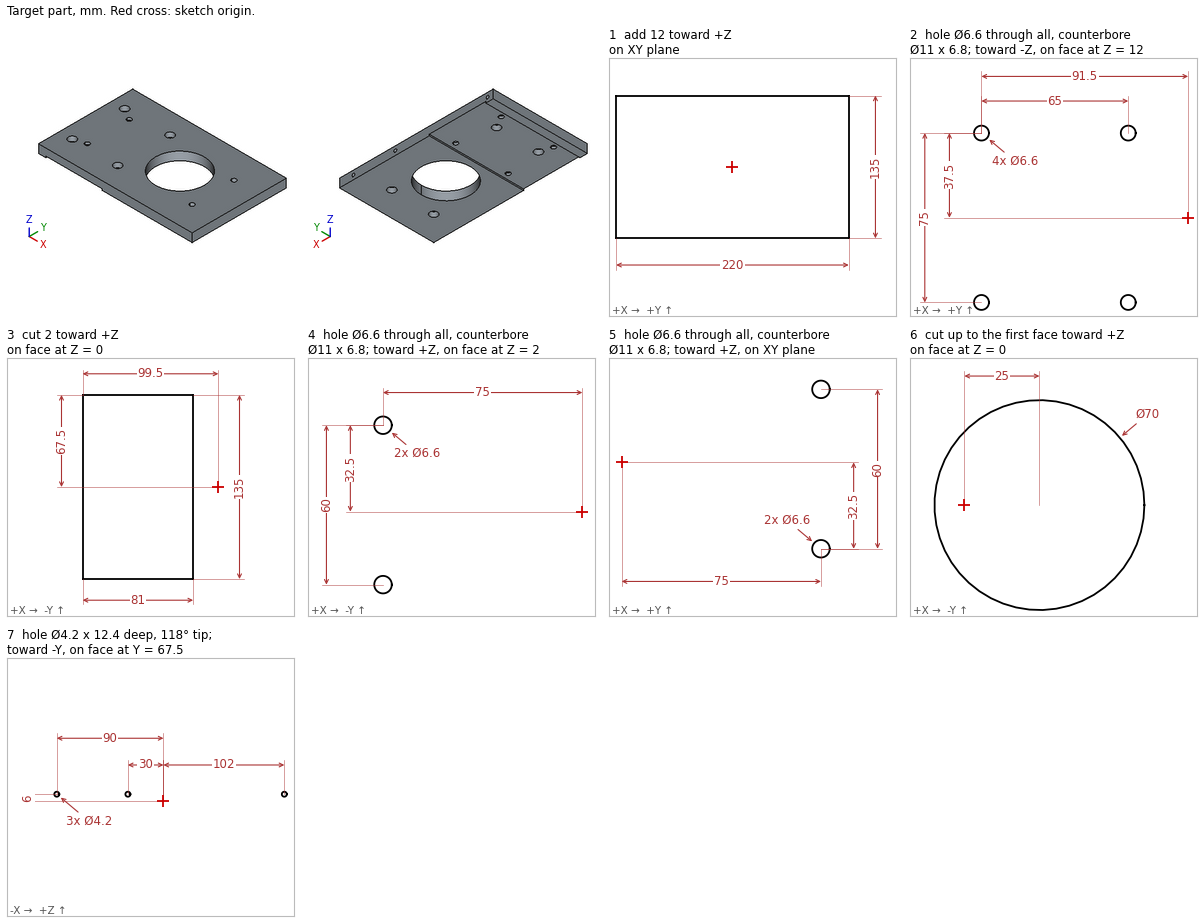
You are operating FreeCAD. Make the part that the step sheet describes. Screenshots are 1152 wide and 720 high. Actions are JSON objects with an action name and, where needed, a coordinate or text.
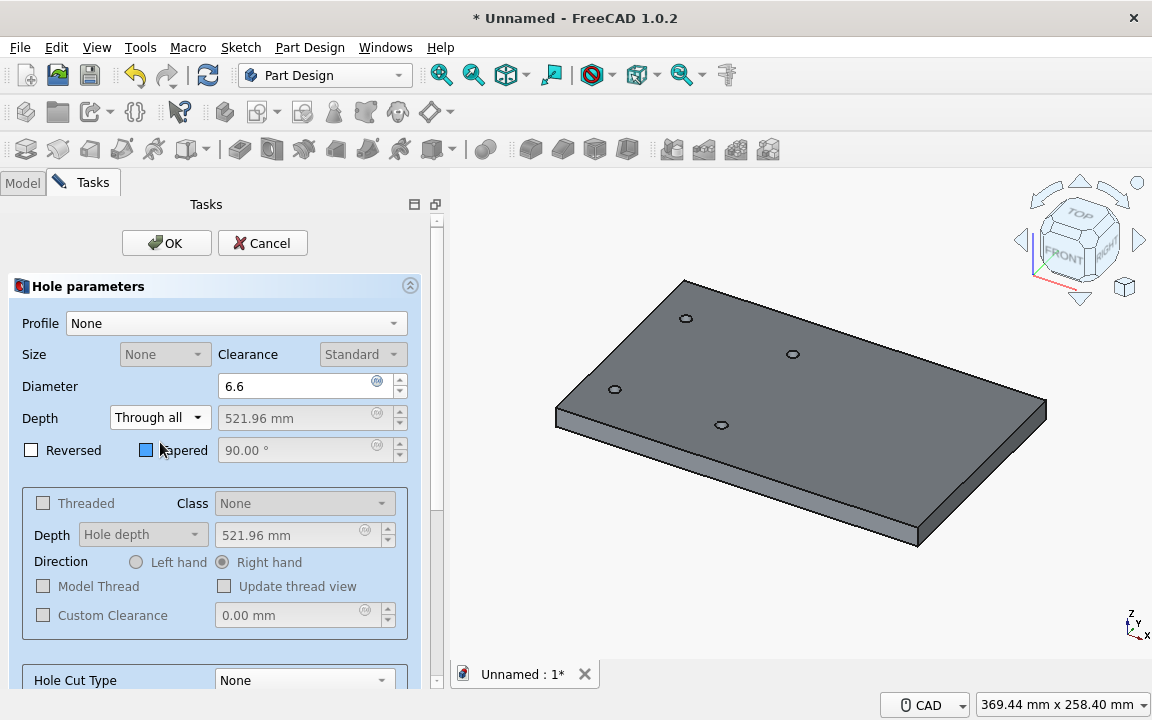
{"action": "scroll", "coordinate": [437, 451], "scroll_direction": "down", "scroll_amount": 2}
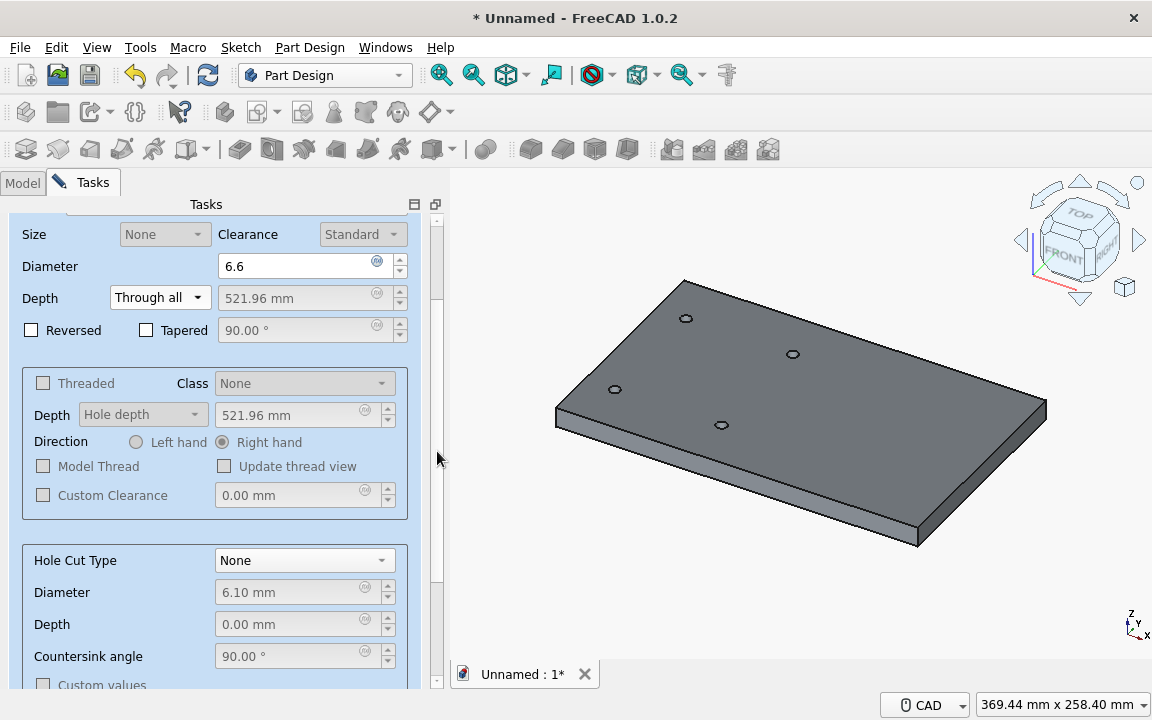
{"action": "left_click", "coordinate": [306, 560]}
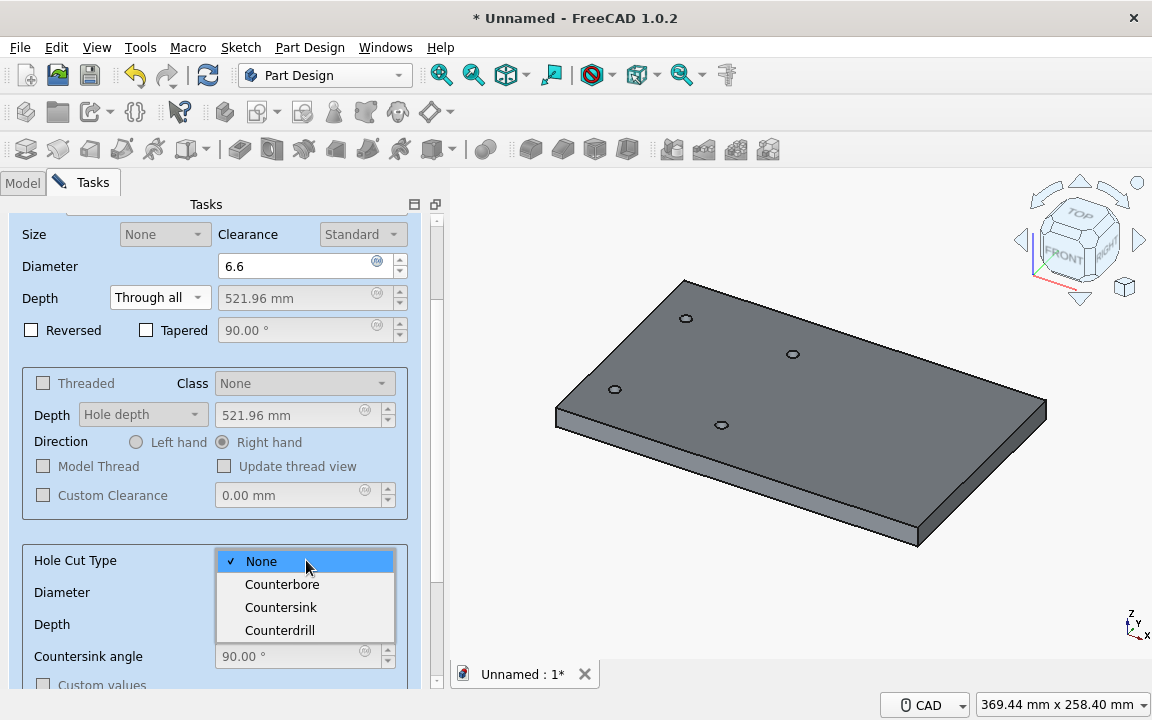
{"action": "left_click", "coordinate": [304, 584]}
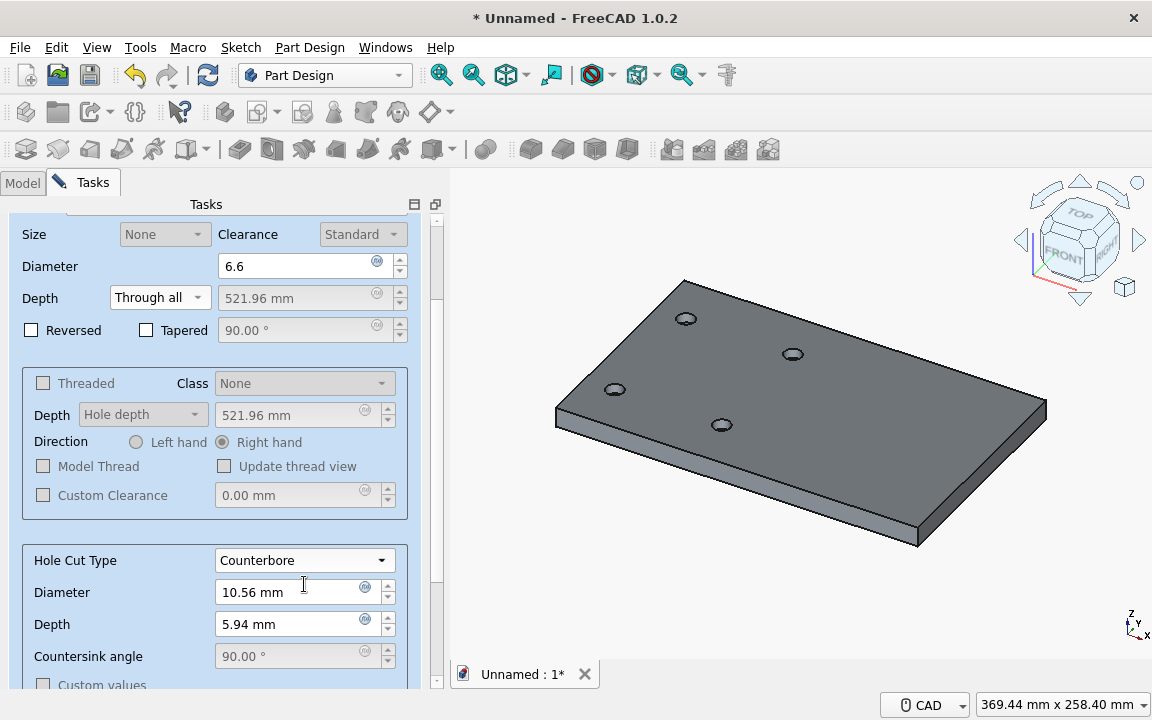
{"action": "triple_click", "coordinate": [298, 592]}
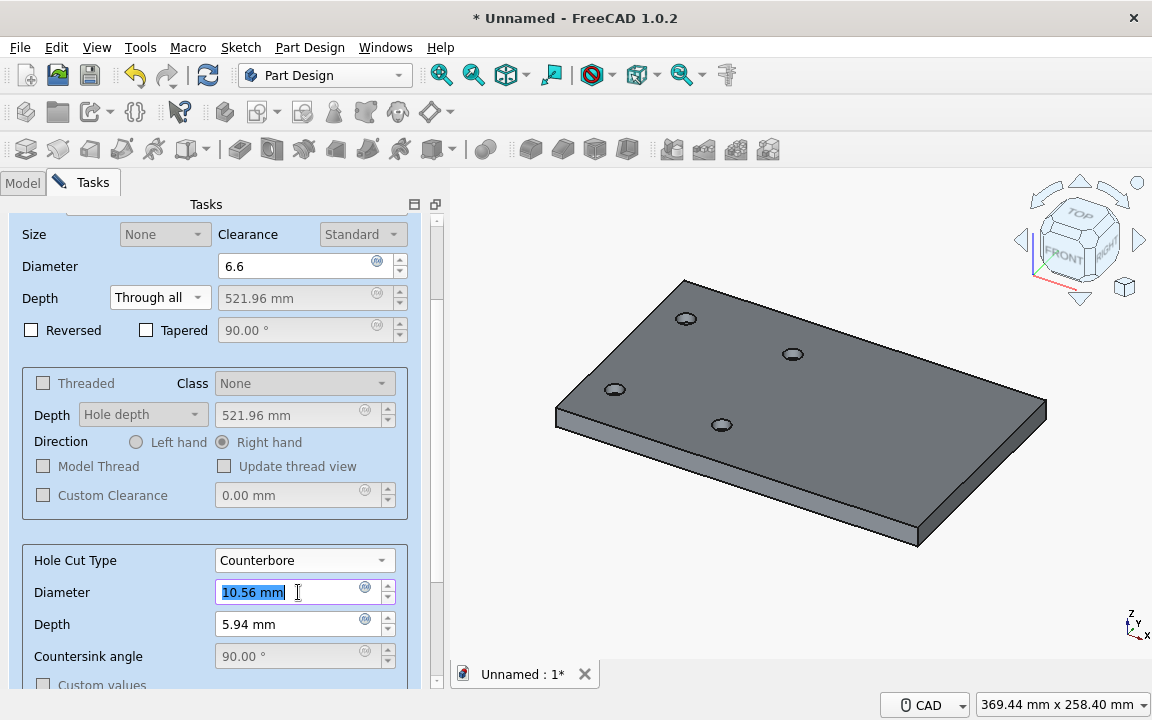
{"action": "type", "text": "11"}
{"action": "key", "text": "Tab"}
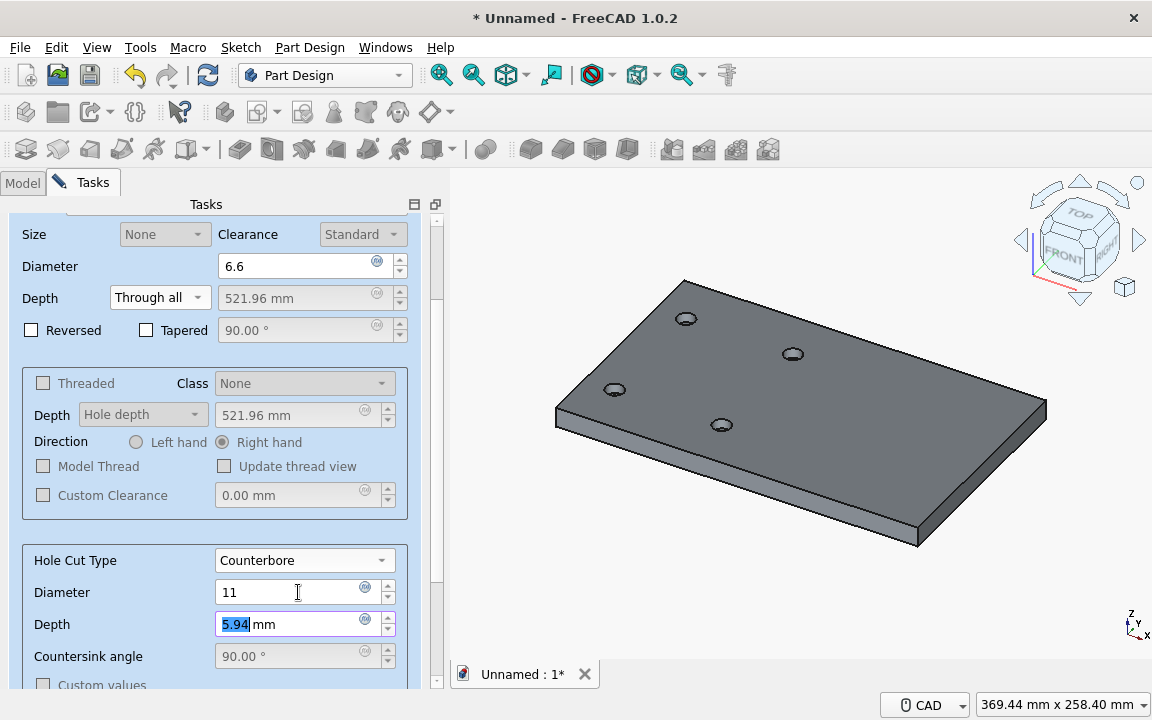
{"action": "type", "text": "6.8"}
{"action": "key", "text": "Tab"}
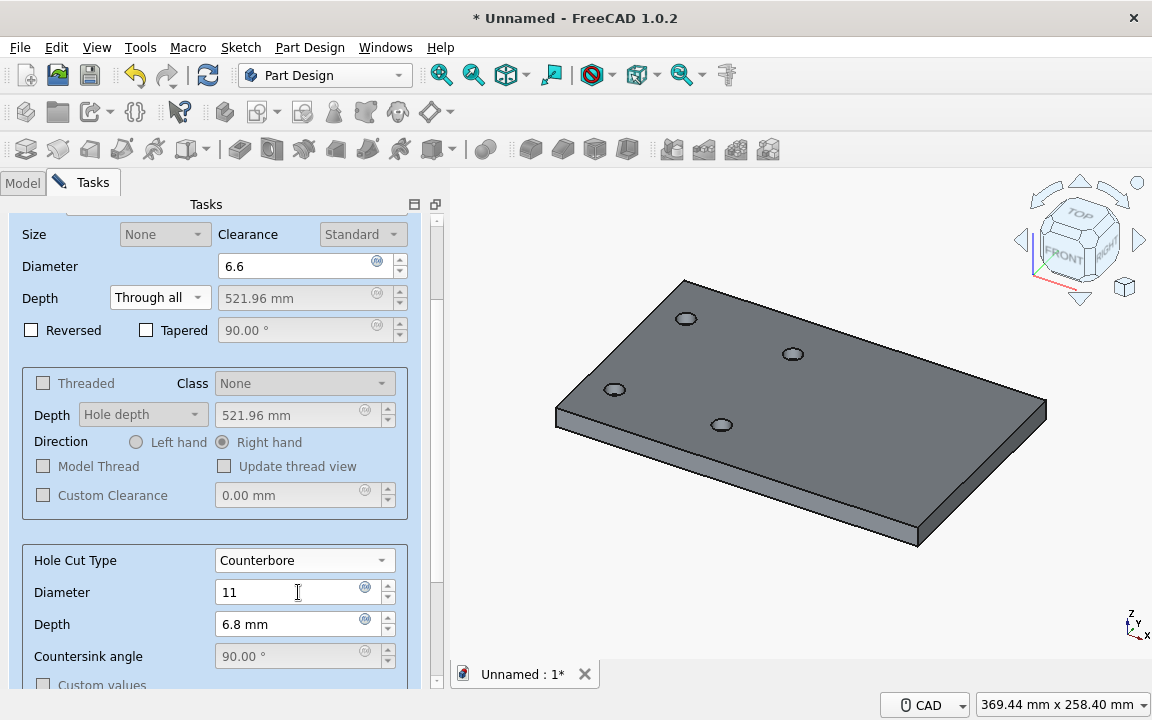
{"action": "scroll", "coordinate": [437, 451], "scroll_direction": "up", "scroll_amount": 3}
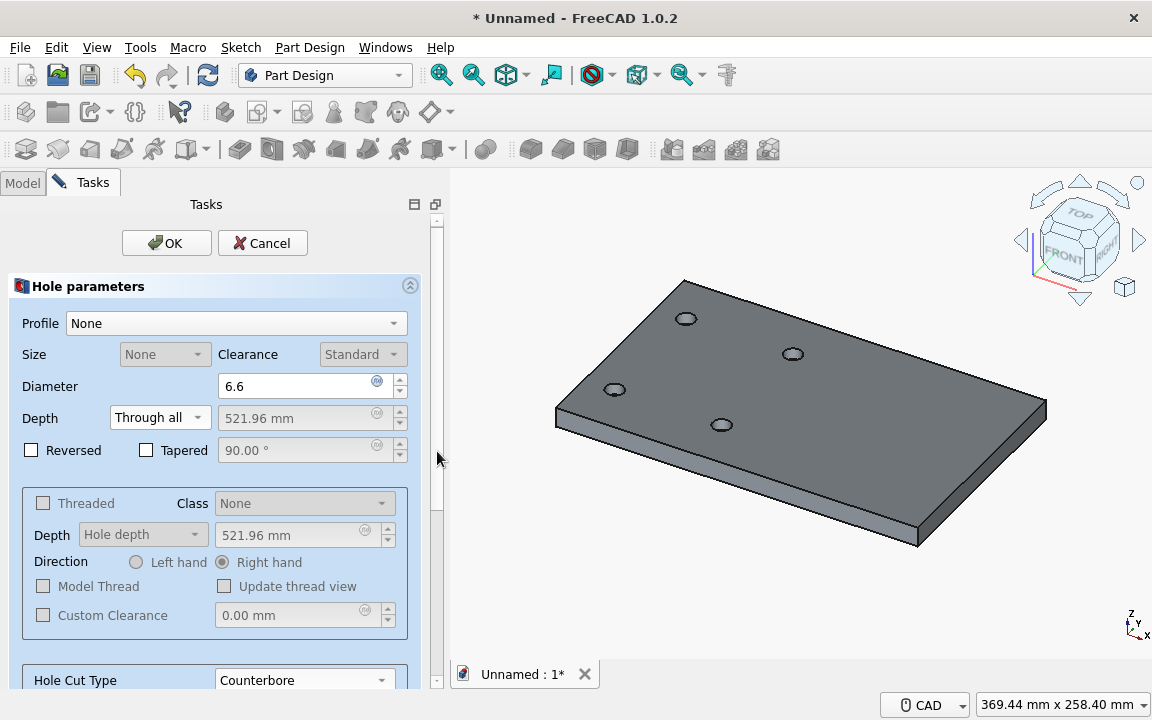
{"action": "left_click", "coordinate": [167, 243]}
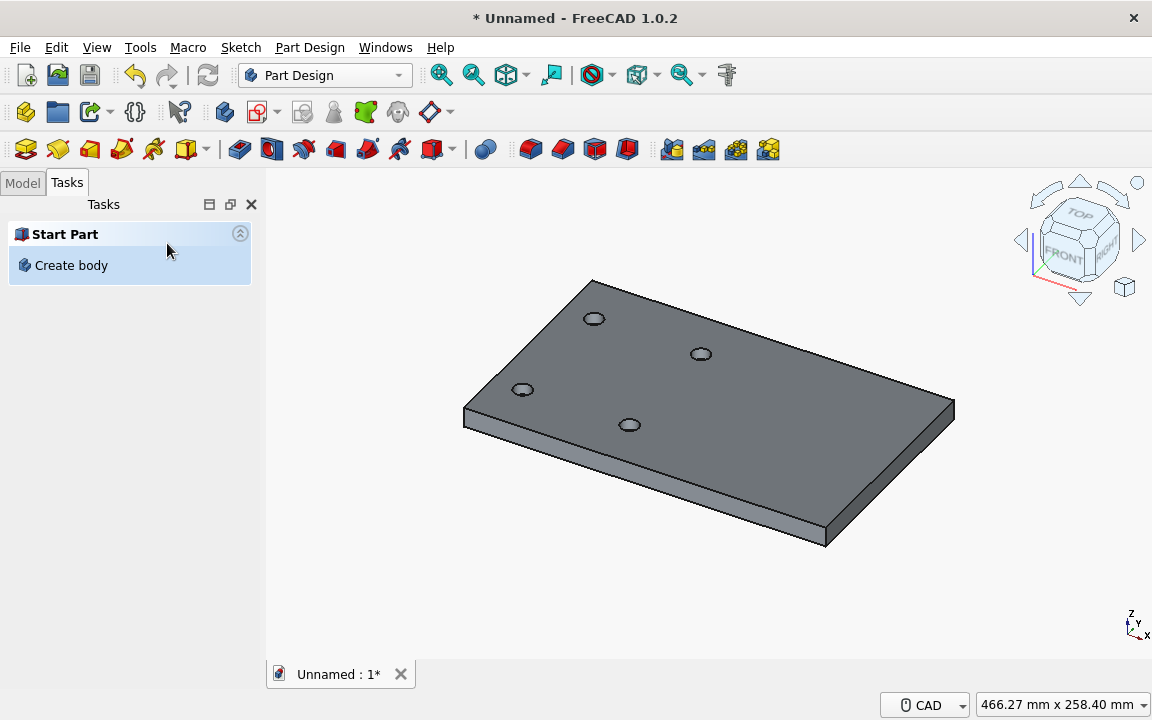
{"action": "key", "text": "5"}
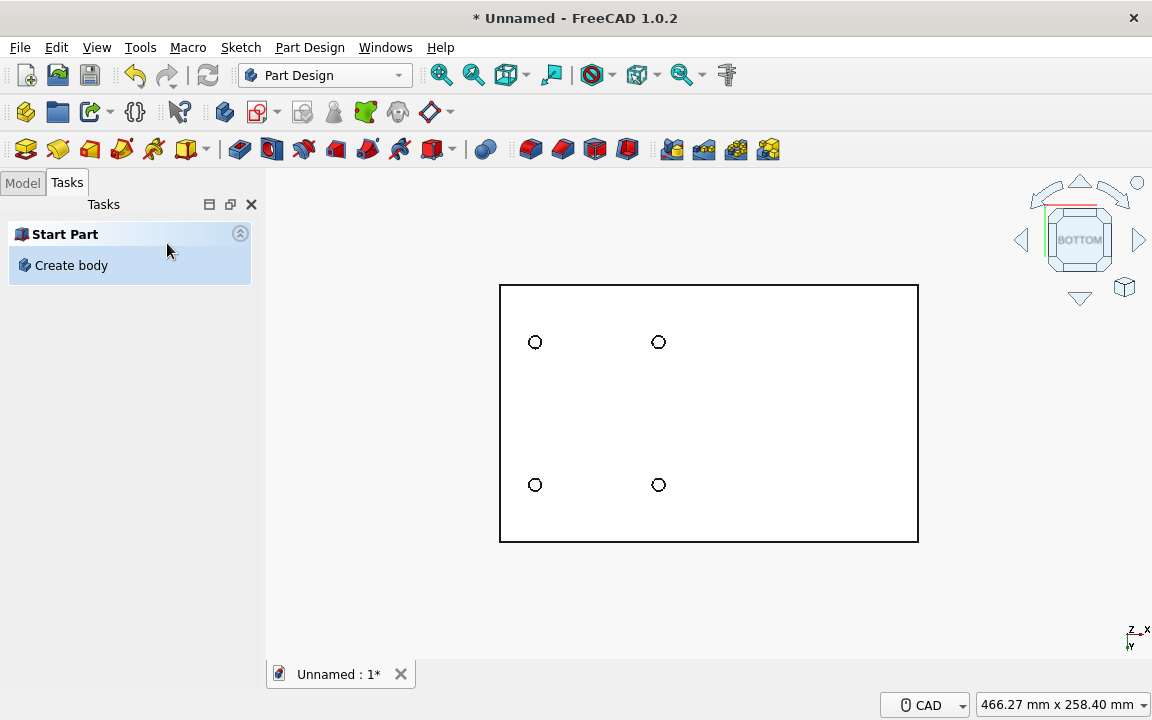
{"action": "left_click", "coordinate": [769, 412]}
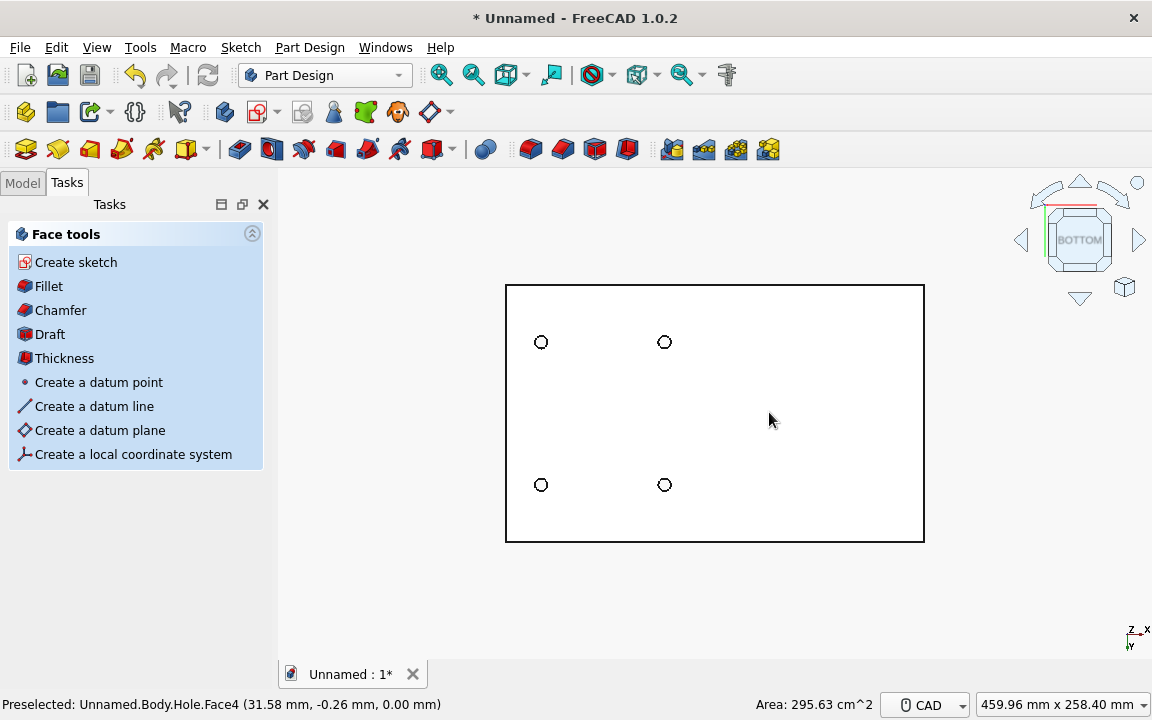
{"action": "left_click", "coordinate": [258, 112]}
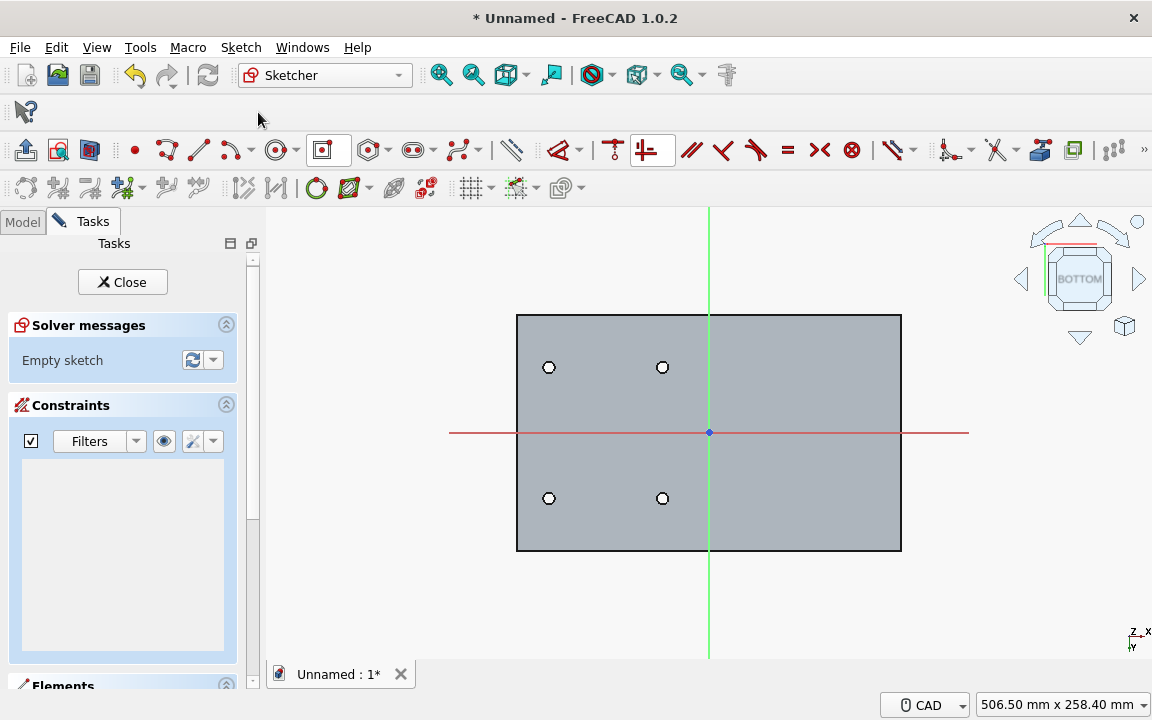
{"action": "key", "text": "g r"}